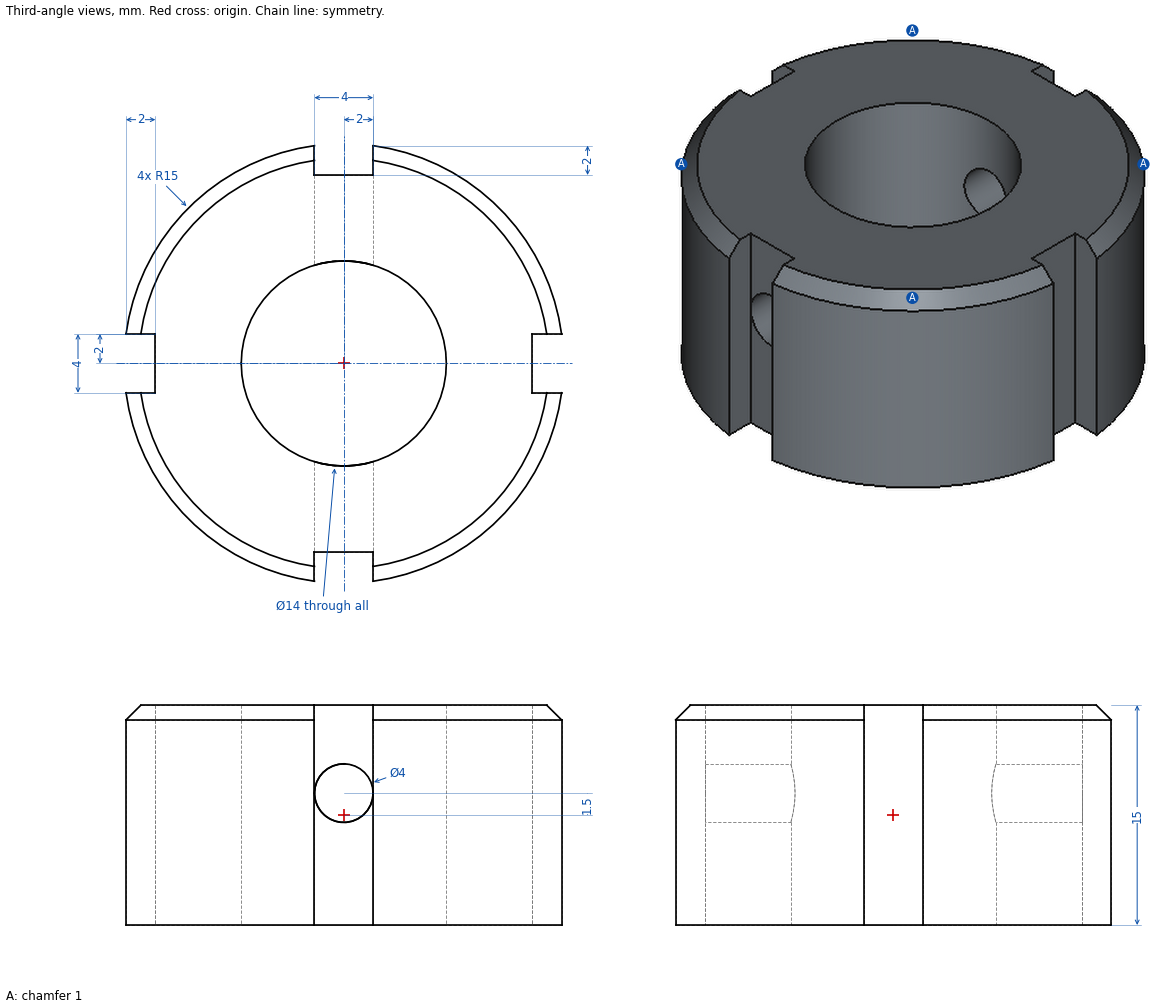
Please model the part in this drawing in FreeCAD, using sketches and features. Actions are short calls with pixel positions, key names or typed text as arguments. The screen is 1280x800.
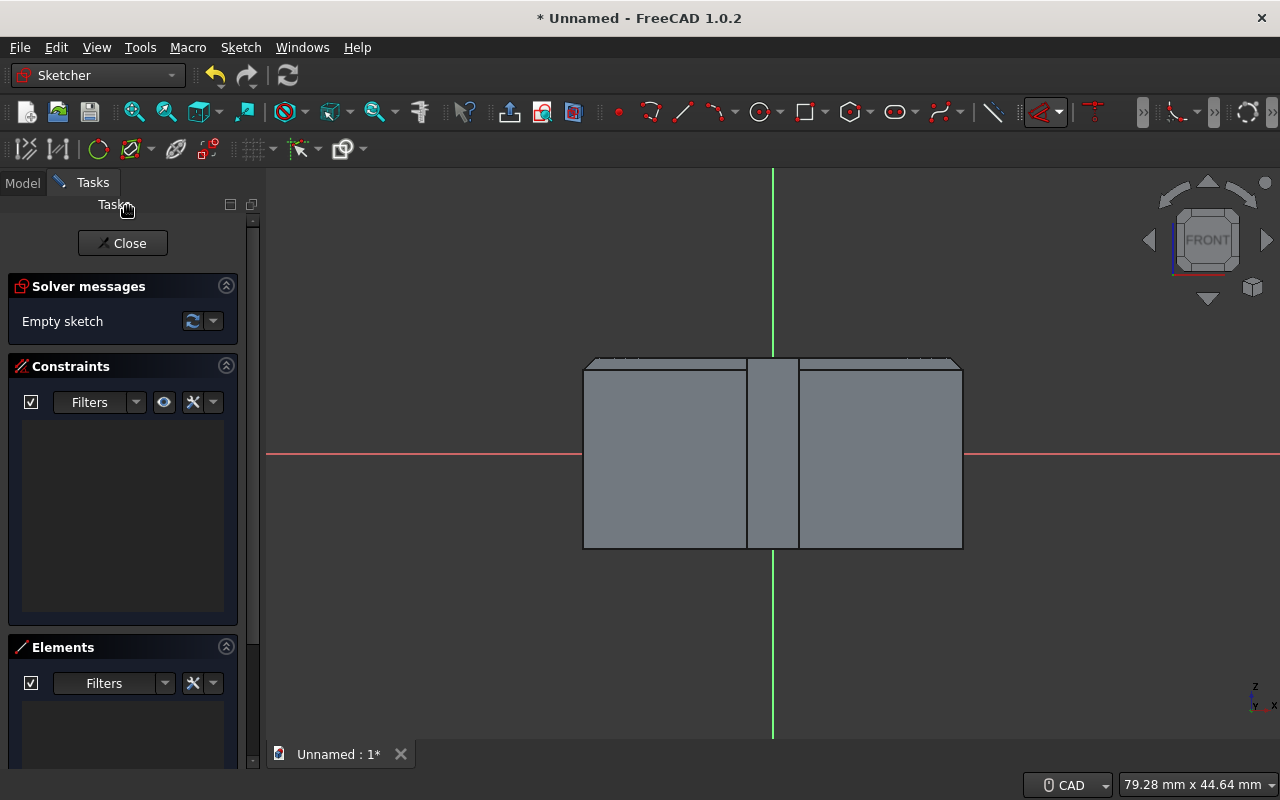
key(q)
key(s)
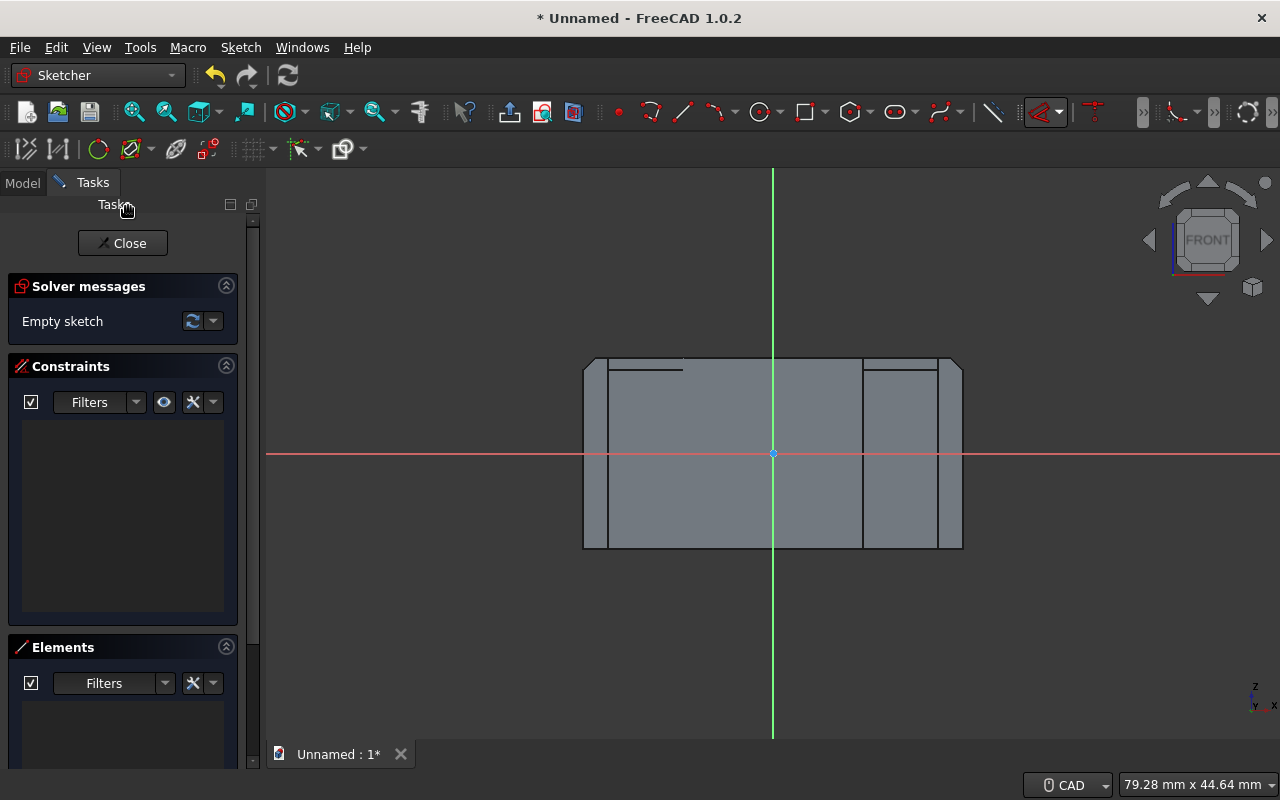
scroll(784, 431, up, 10)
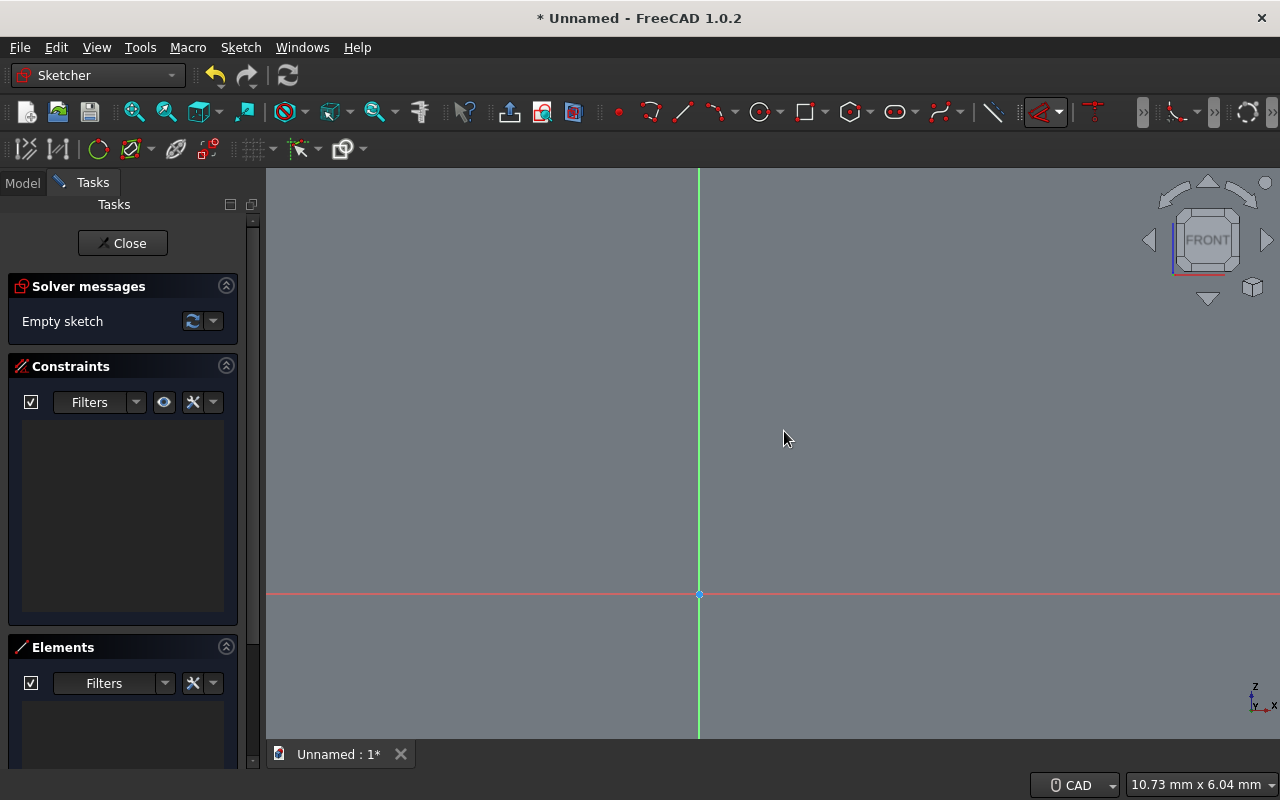
key(g)
key(c)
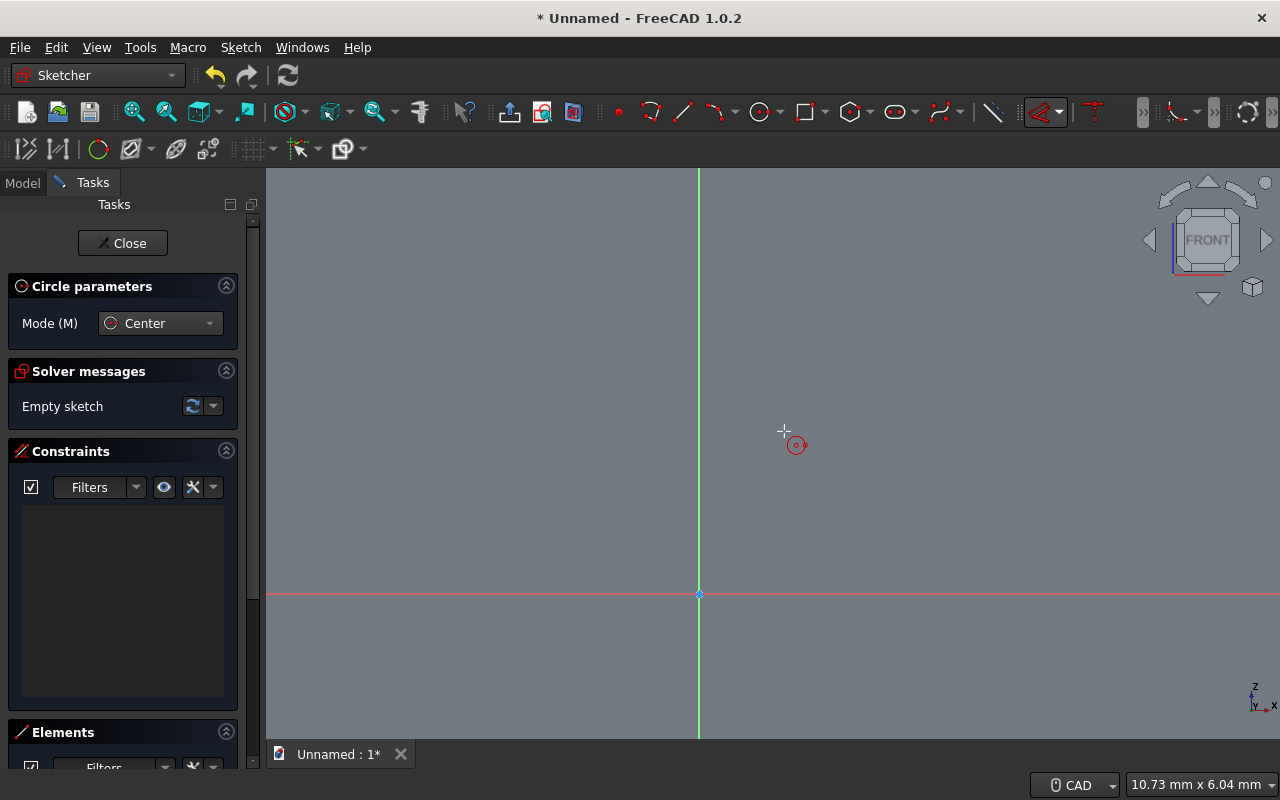
click(699, 453)
move(833, 319)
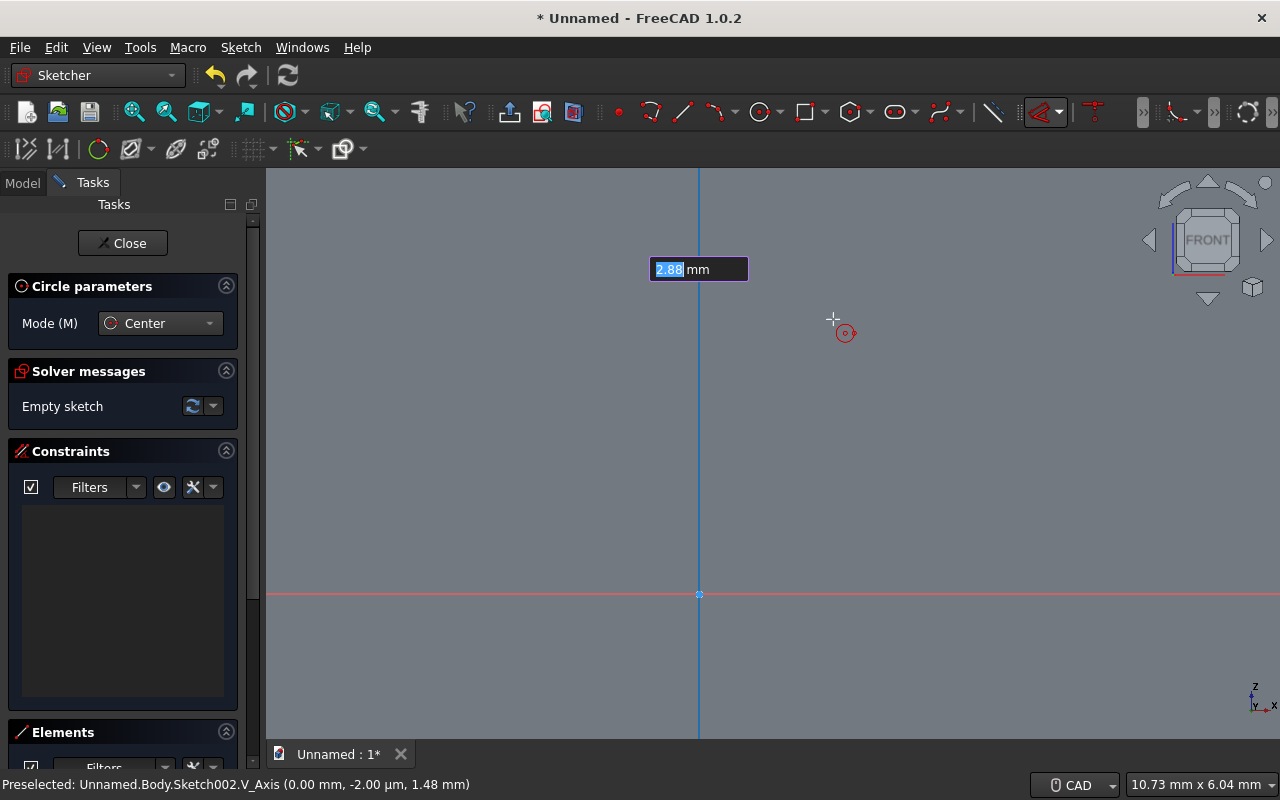
text(4)
key(Return)
key(Escape)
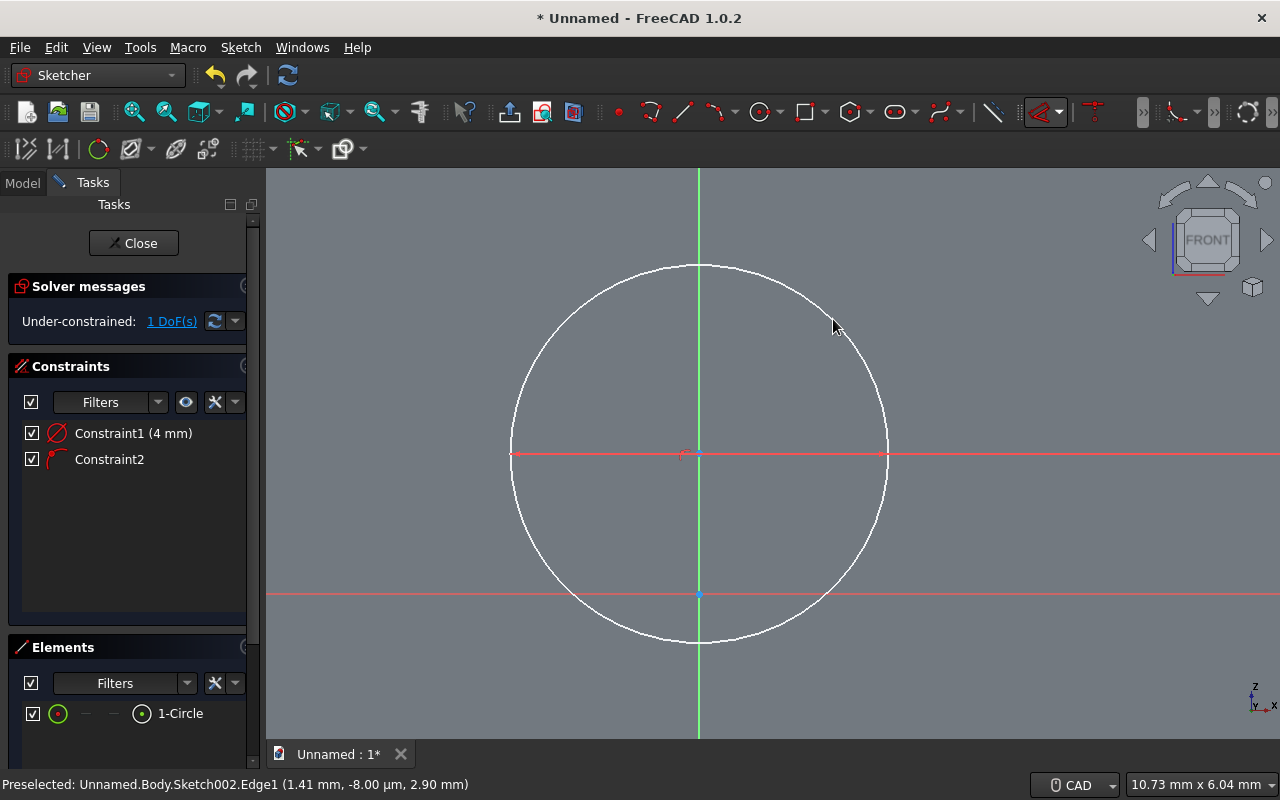
click(699, 454)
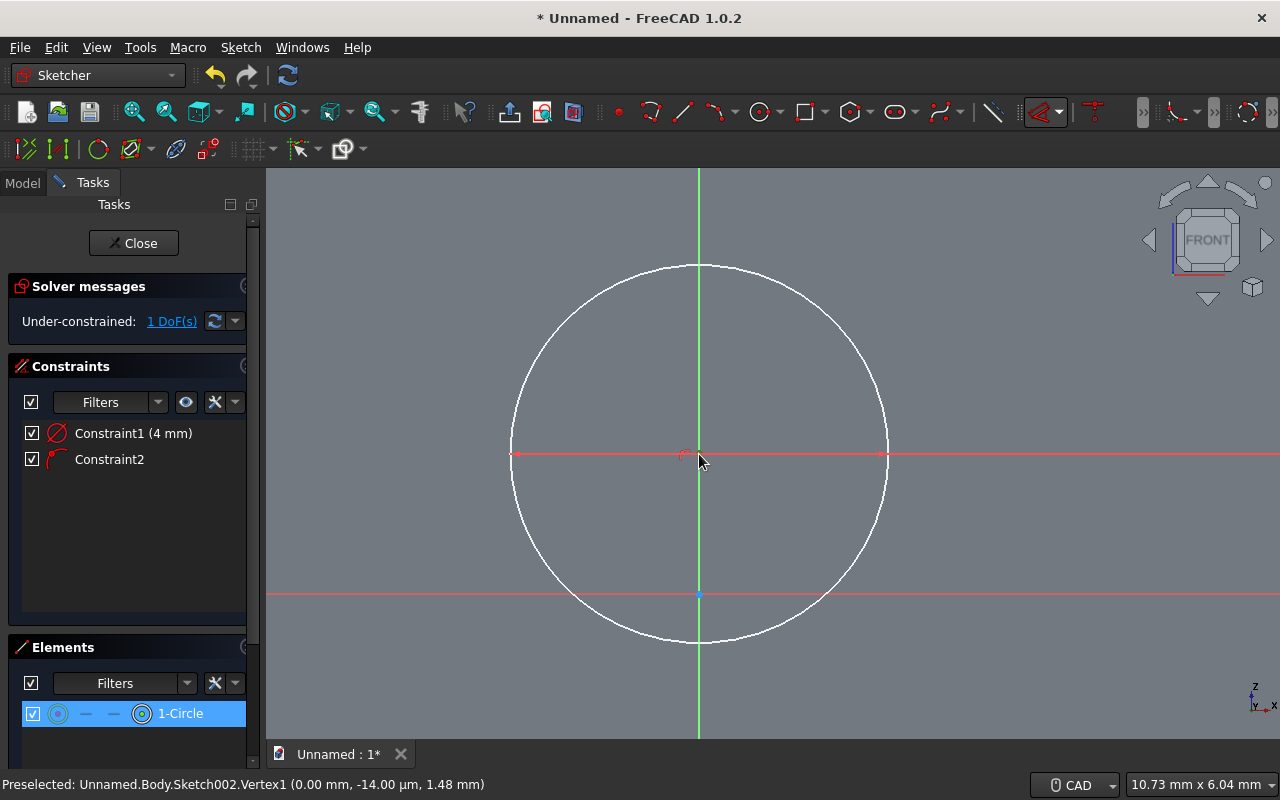
key(i)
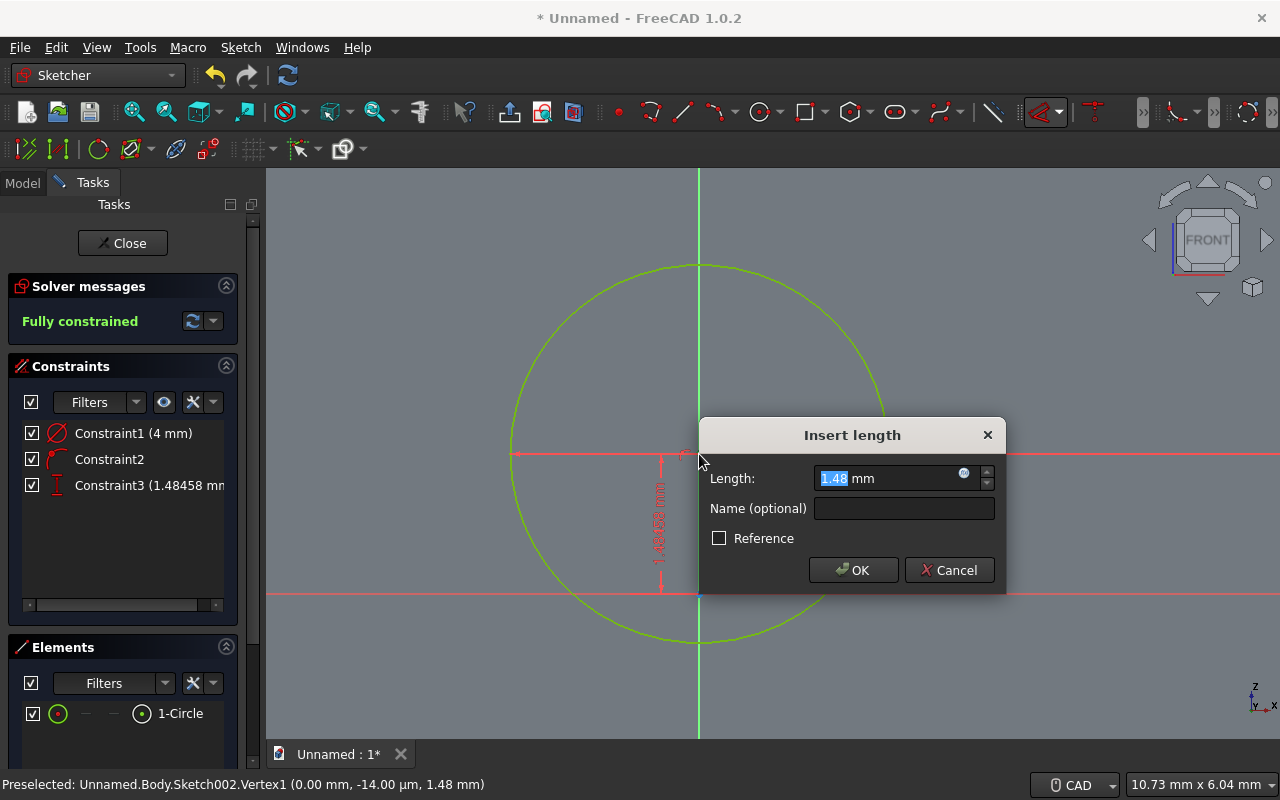
text(1.5)
key(Return)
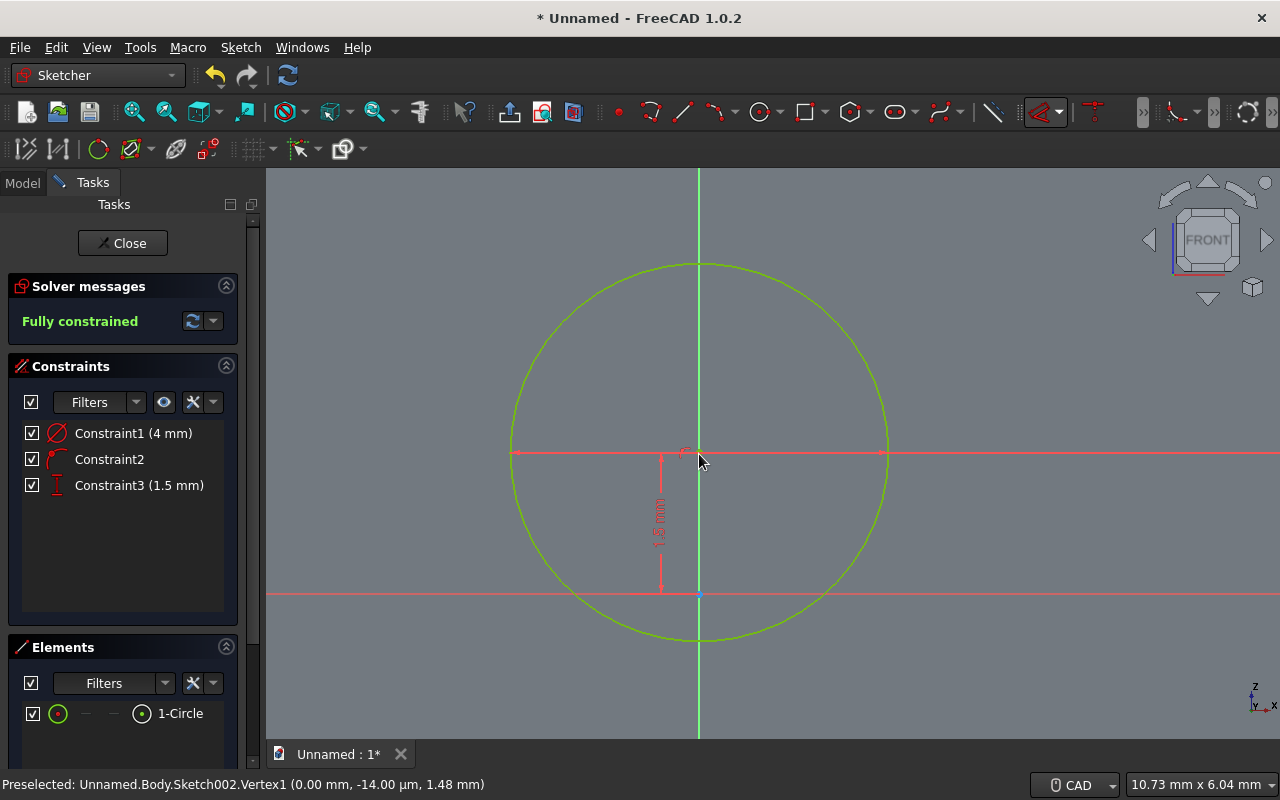
click(123, 243)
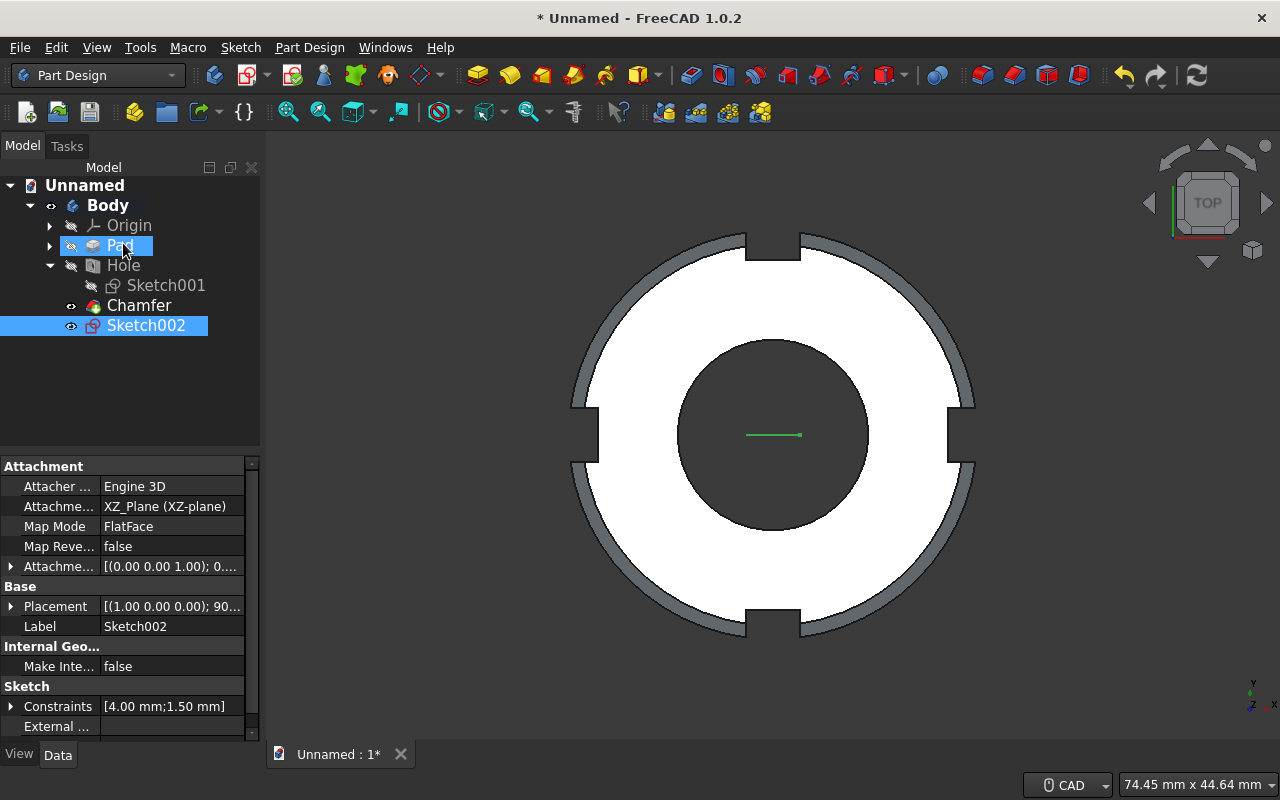
click(692, 76)